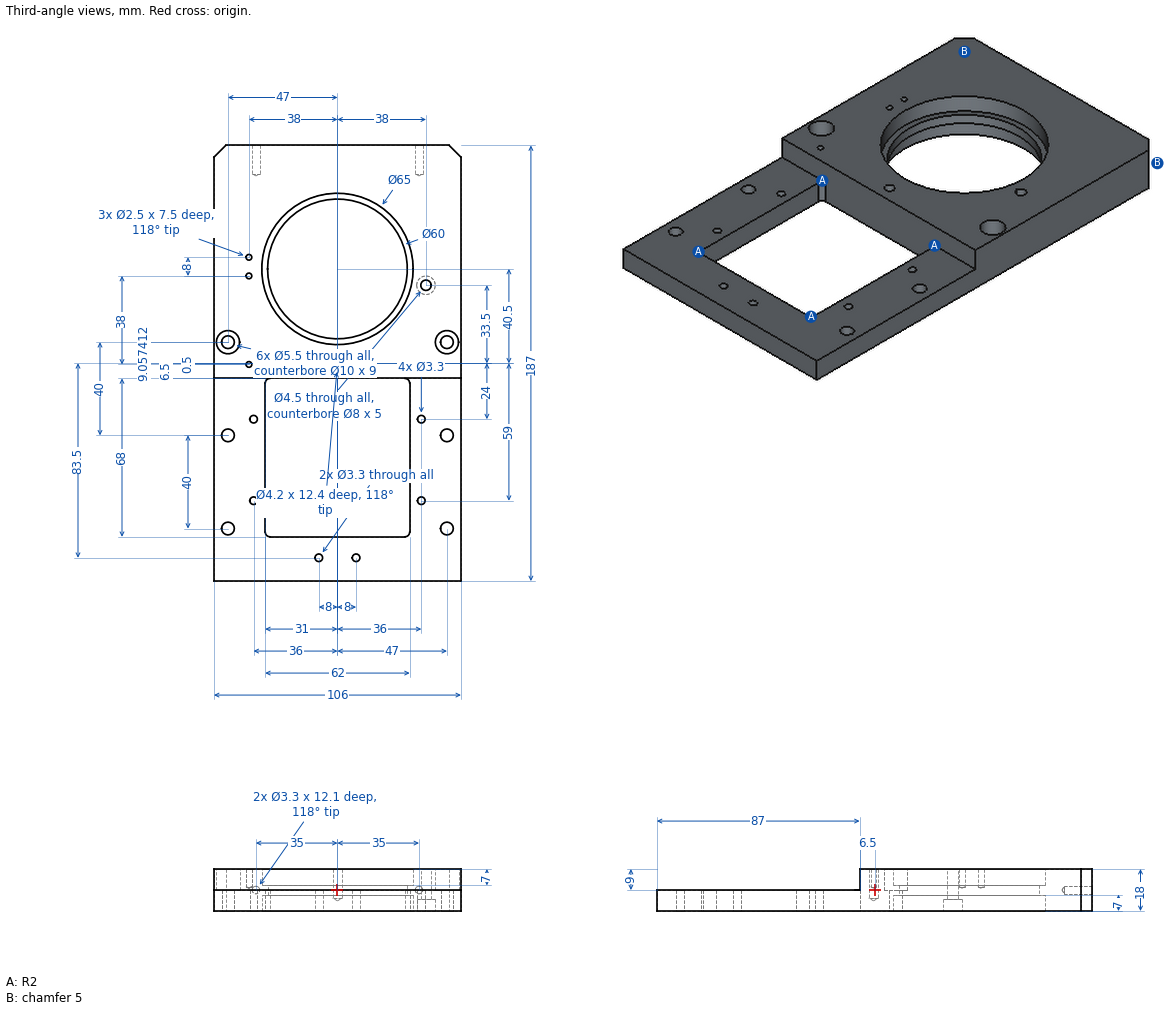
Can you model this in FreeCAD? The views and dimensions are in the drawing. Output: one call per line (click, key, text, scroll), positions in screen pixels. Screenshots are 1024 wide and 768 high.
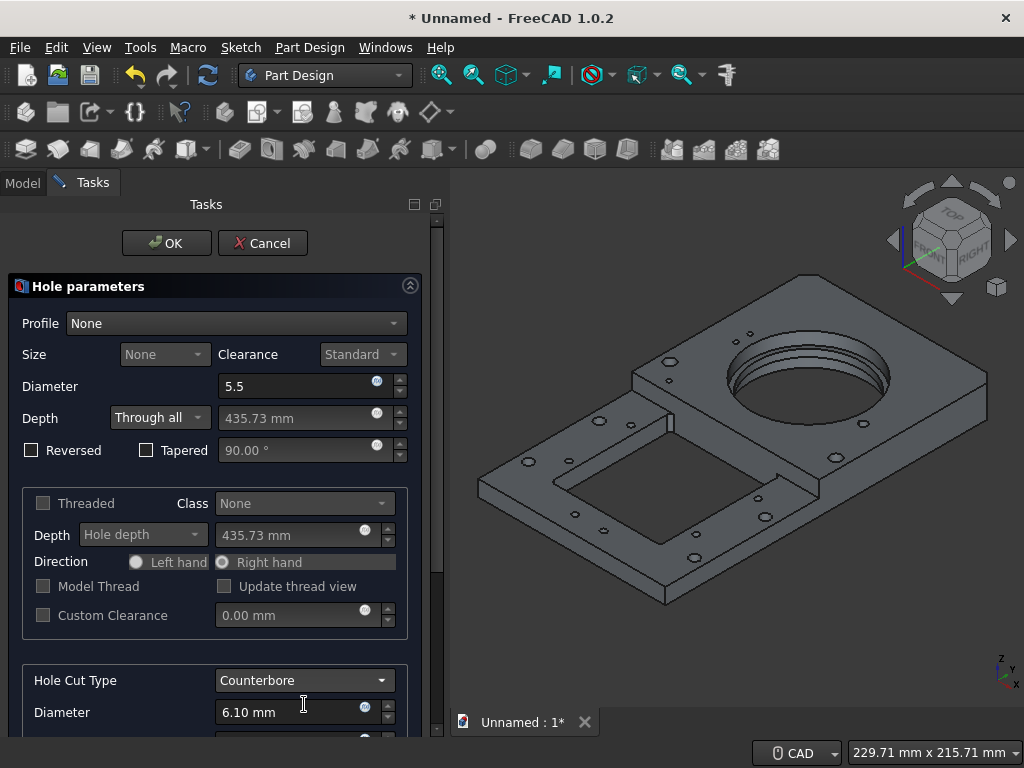
triple_click(298, 712)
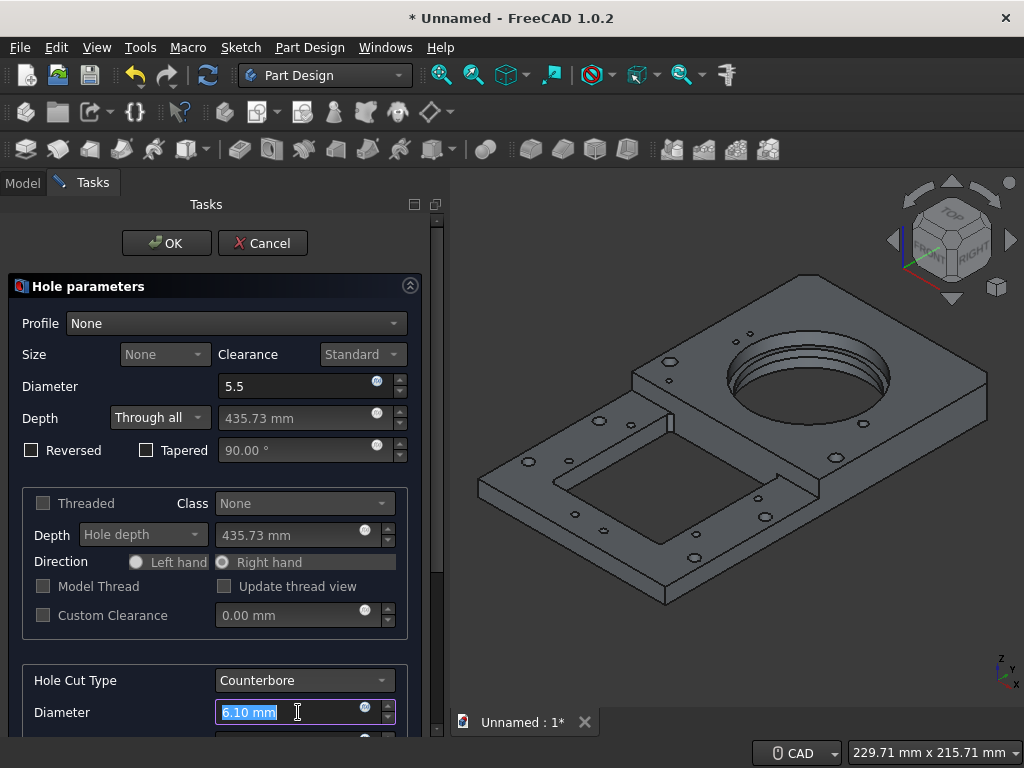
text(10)
key(Tab)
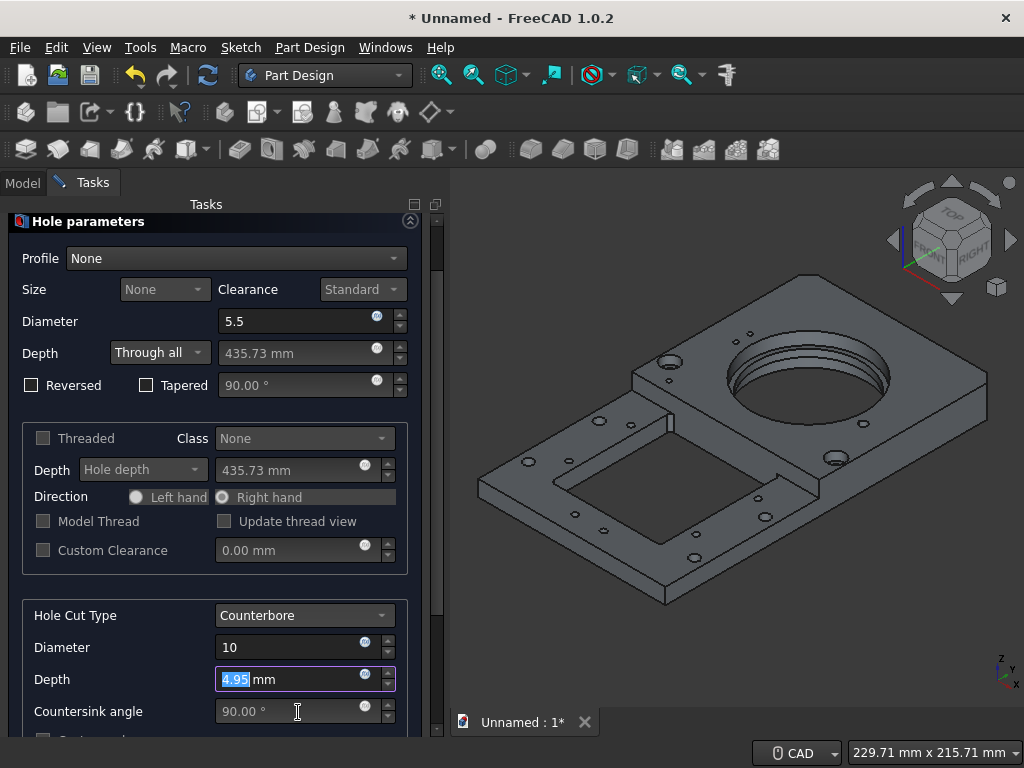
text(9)
key(Tab)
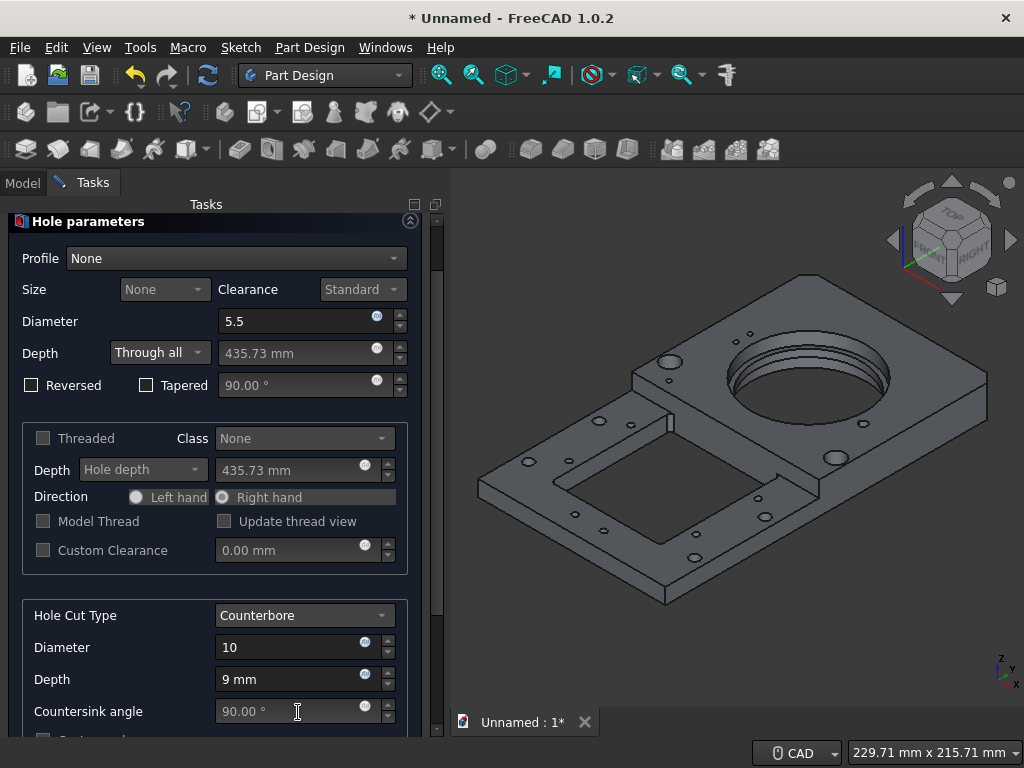
scroll(437, 475, up, 2)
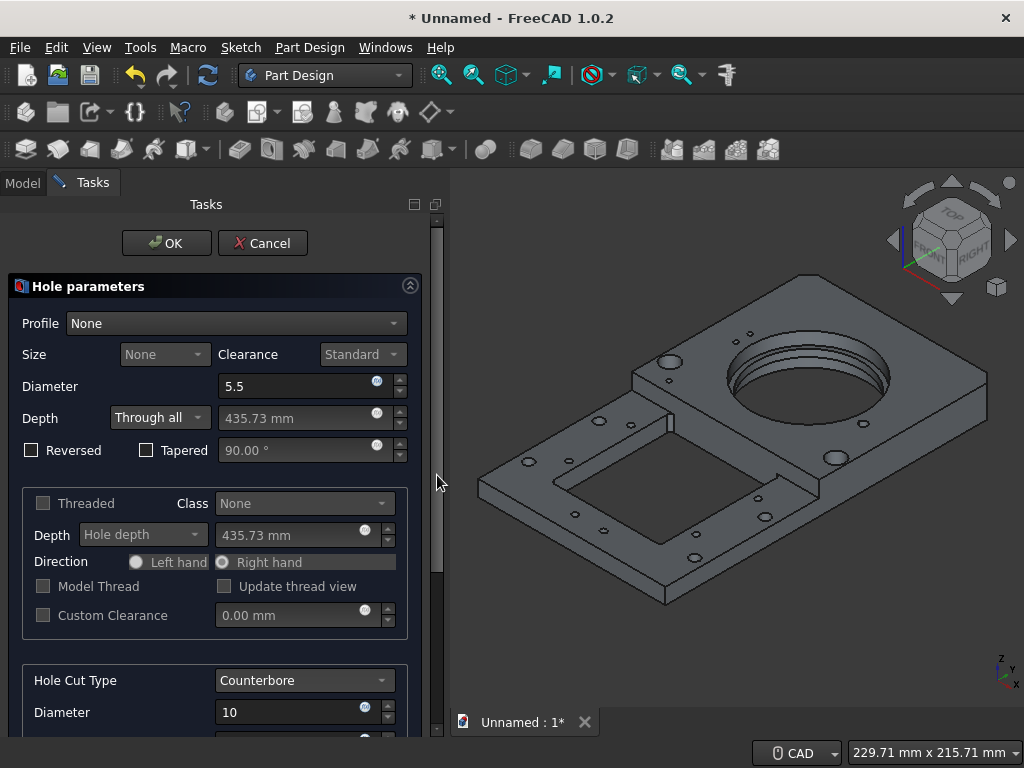
click(167, 243)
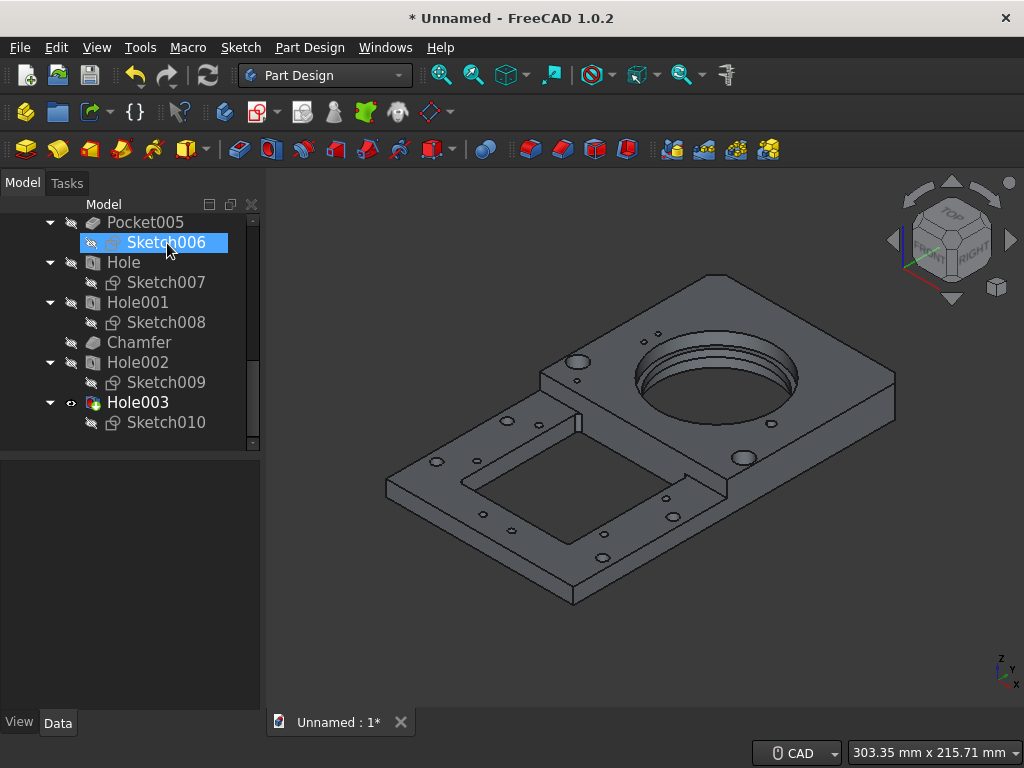
click(826, 376)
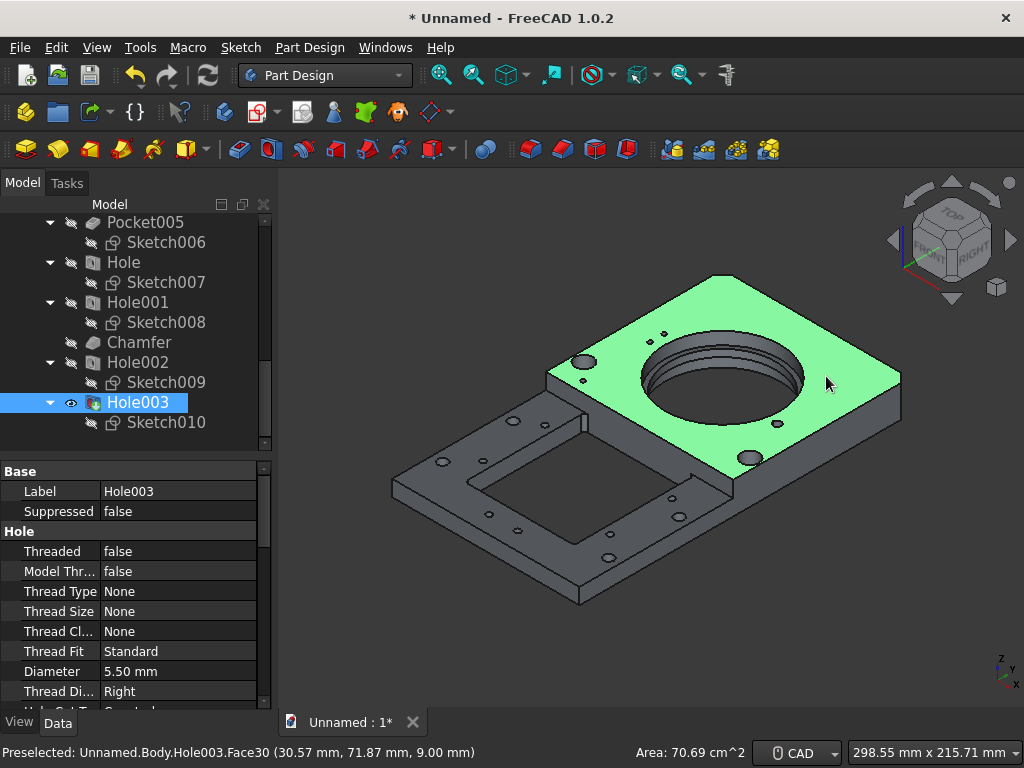
click(258, 112)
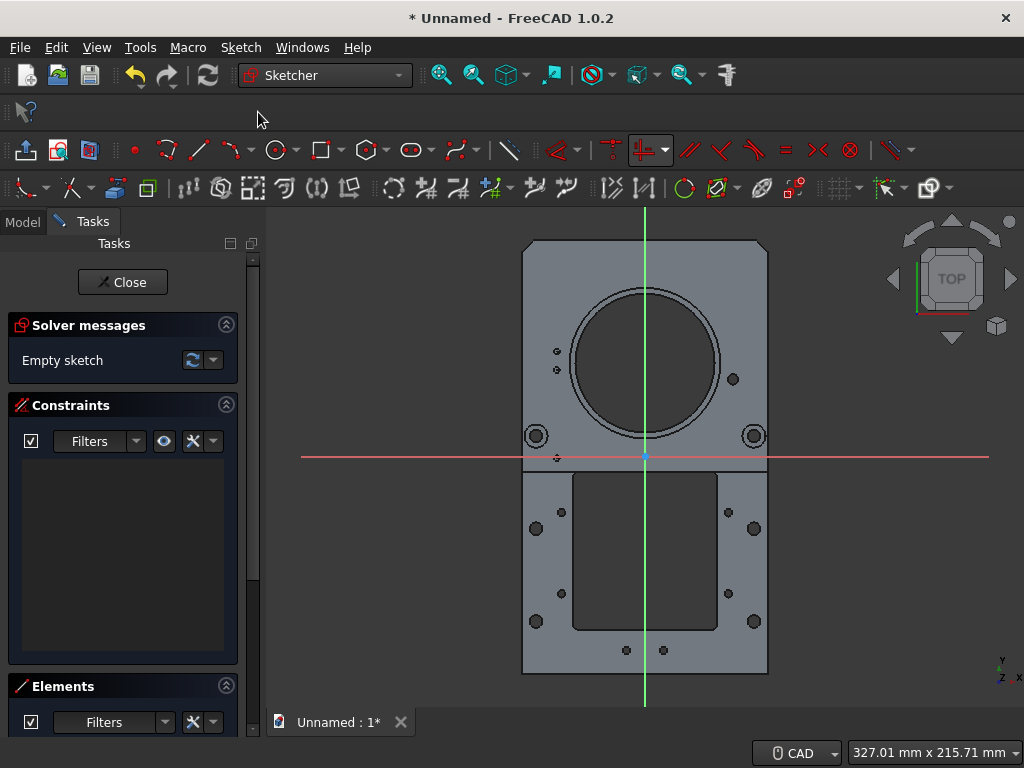
scroll(649, 458, up, 15)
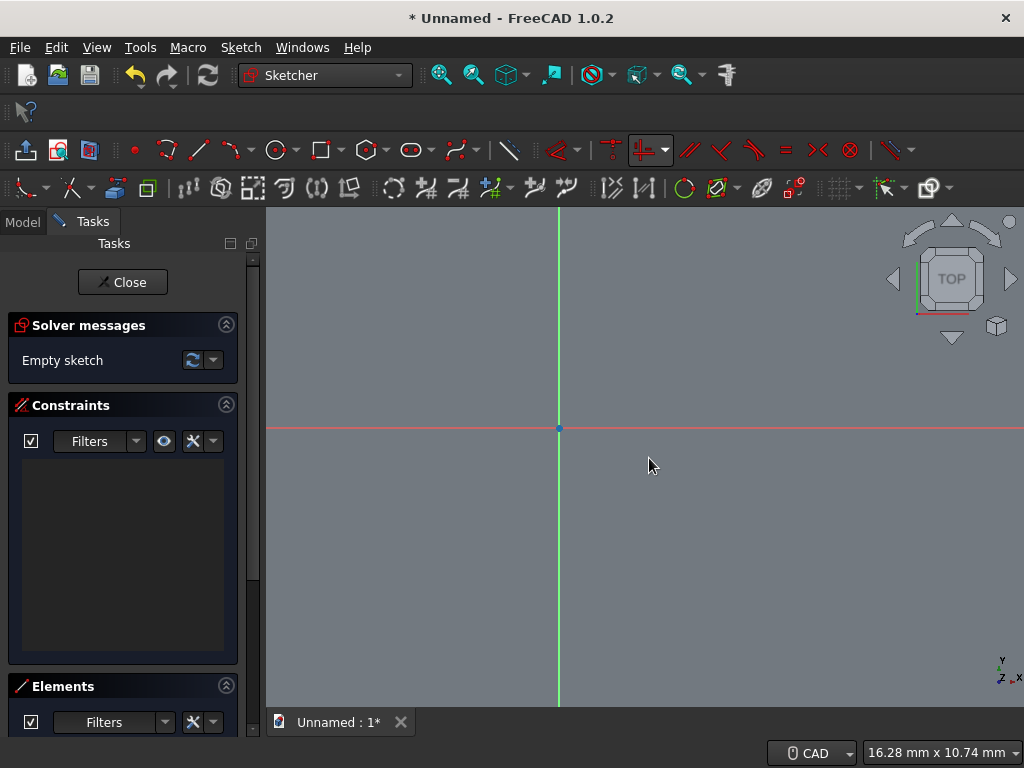
scroll(523, 441, up, 2)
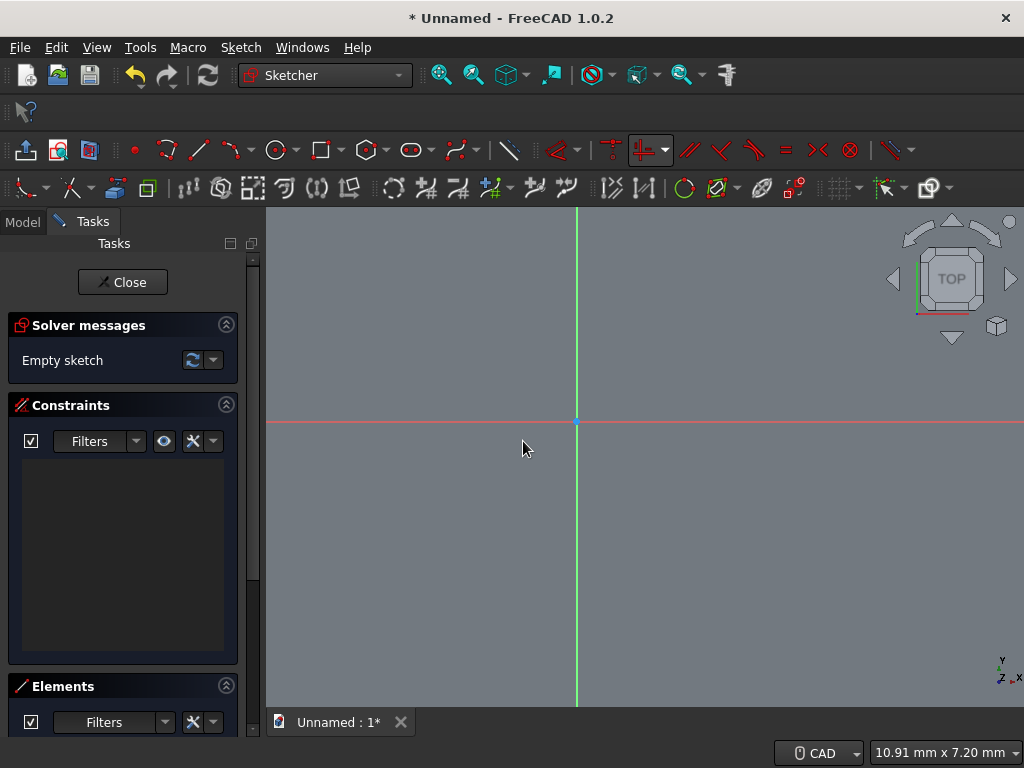
click(276, 150)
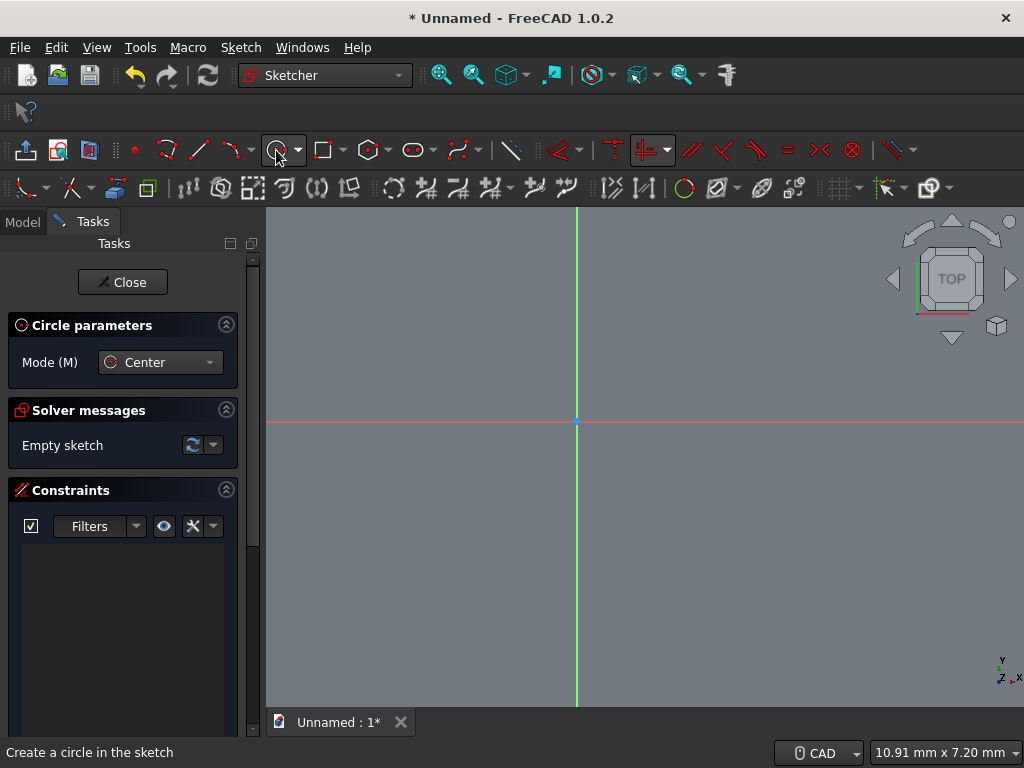
click(577, 457)
click(680, 353)
key(Escape)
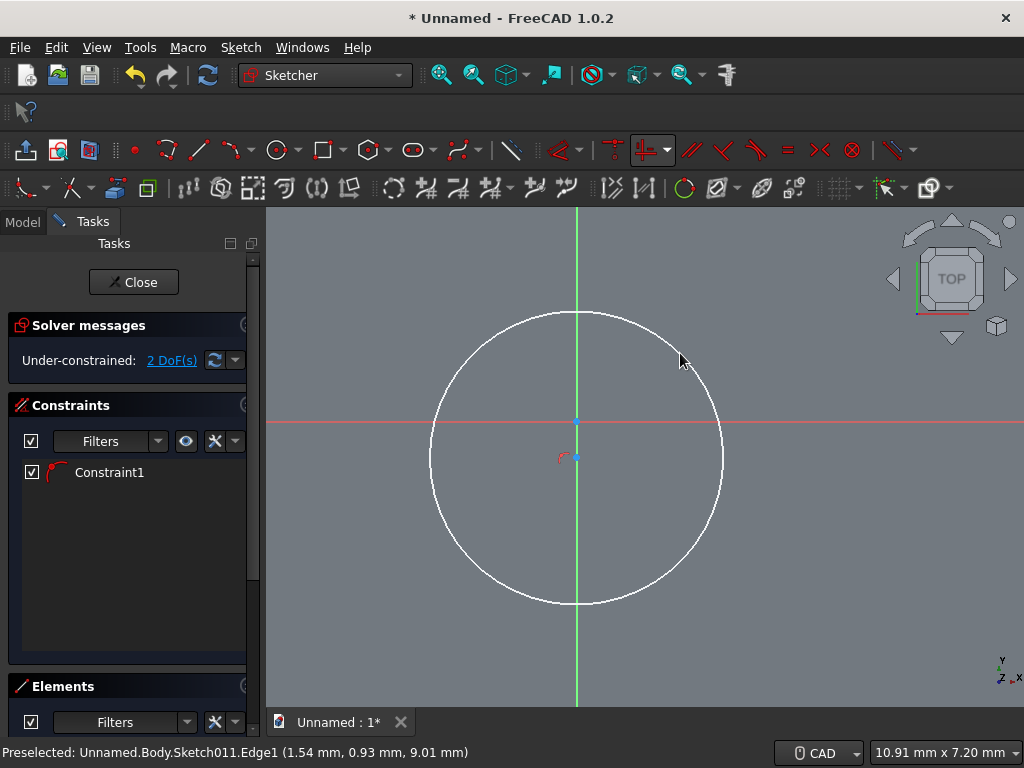
click(558, 150)